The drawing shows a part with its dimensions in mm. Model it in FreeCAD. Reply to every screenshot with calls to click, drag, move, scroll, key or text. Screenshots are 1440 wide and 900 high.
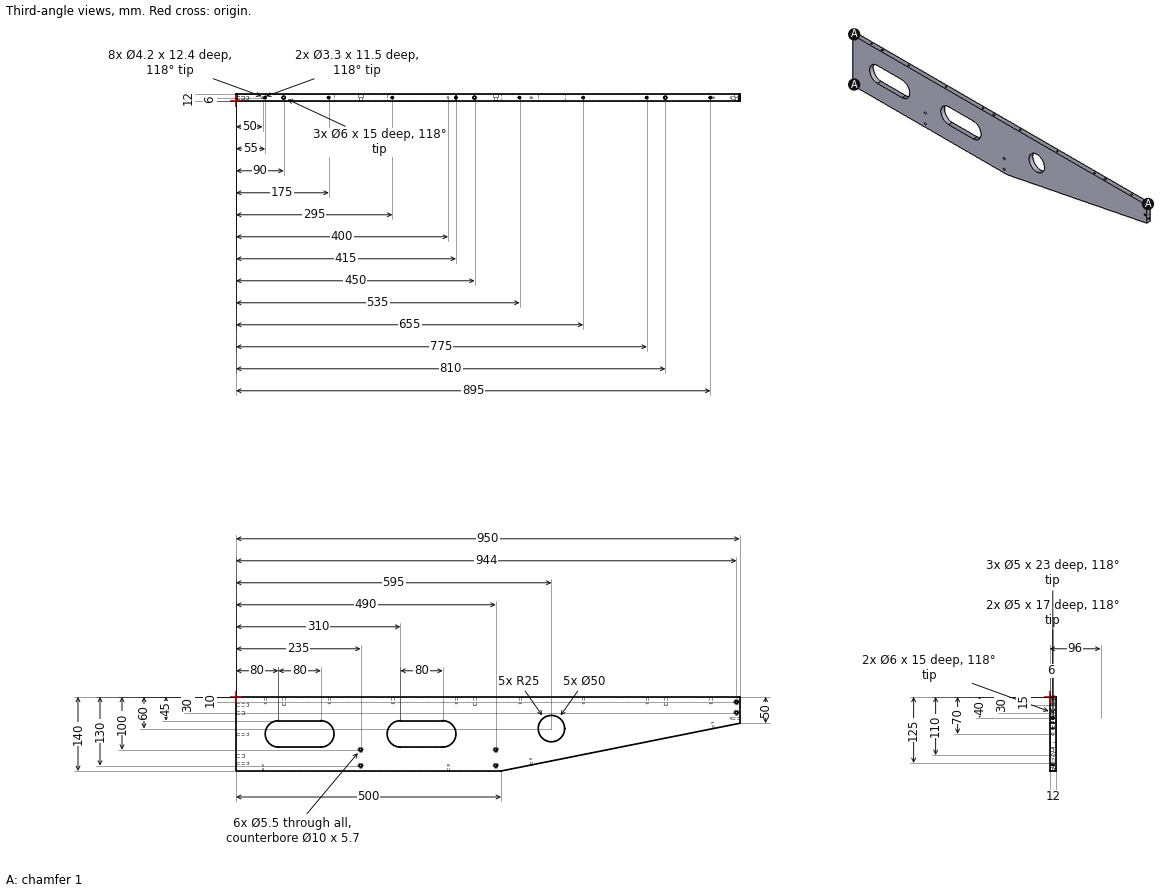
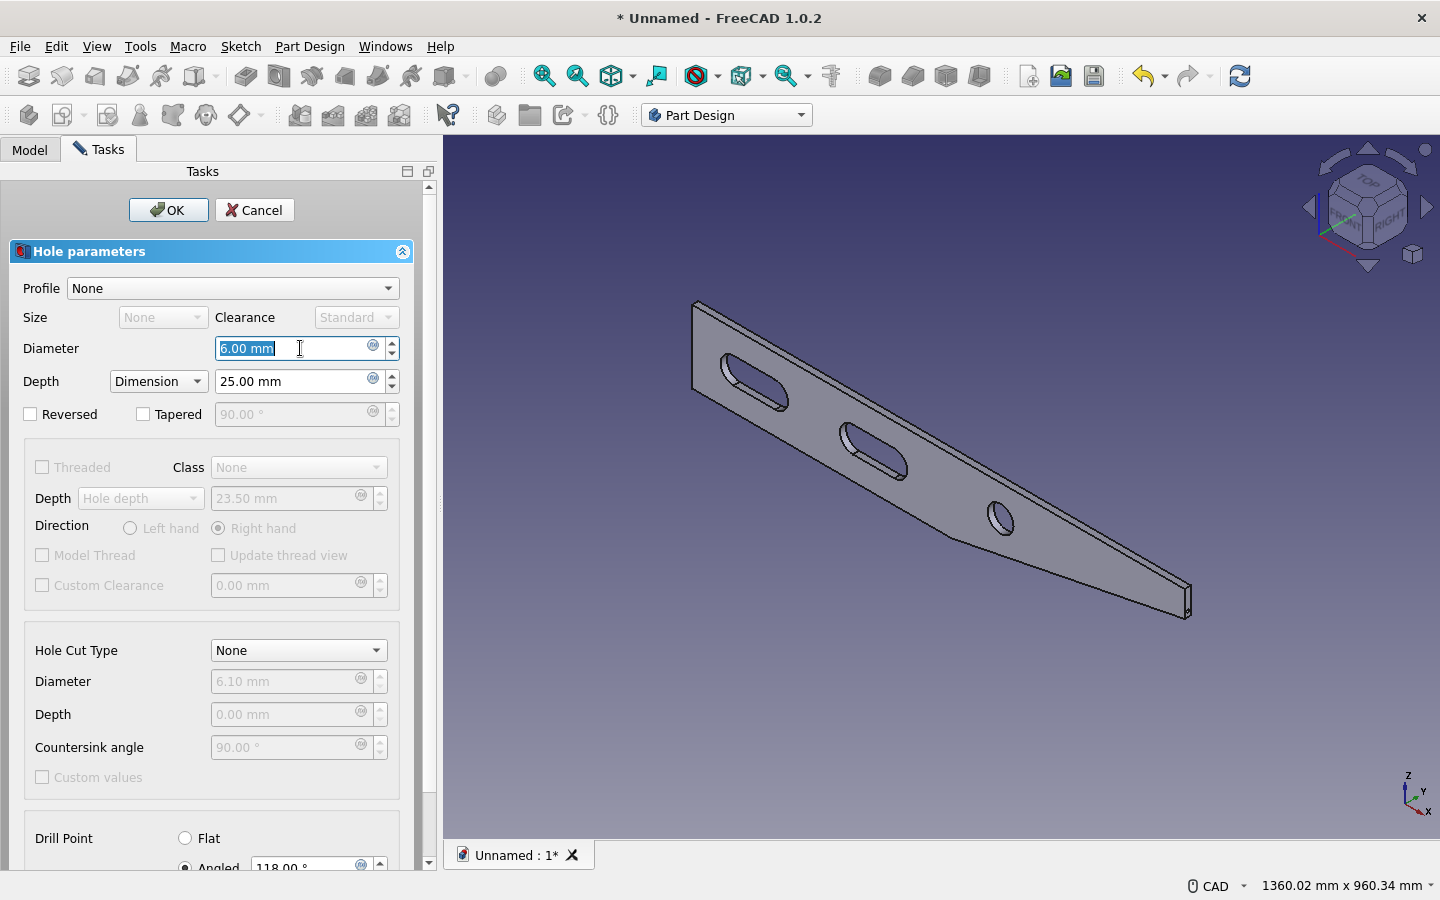
text(5)
key(Tab)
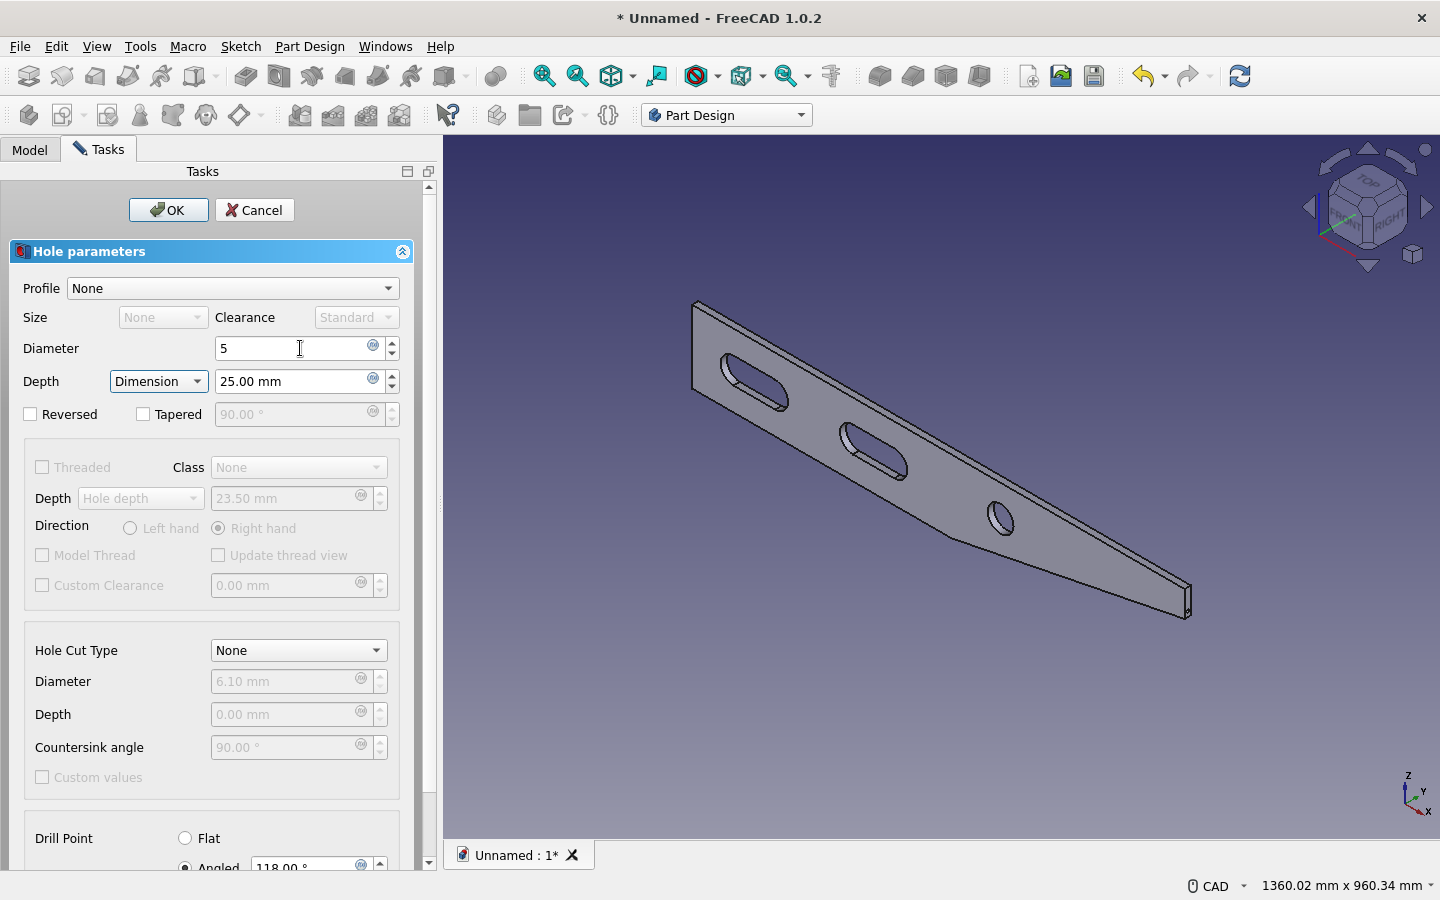
triple_click(300, 382)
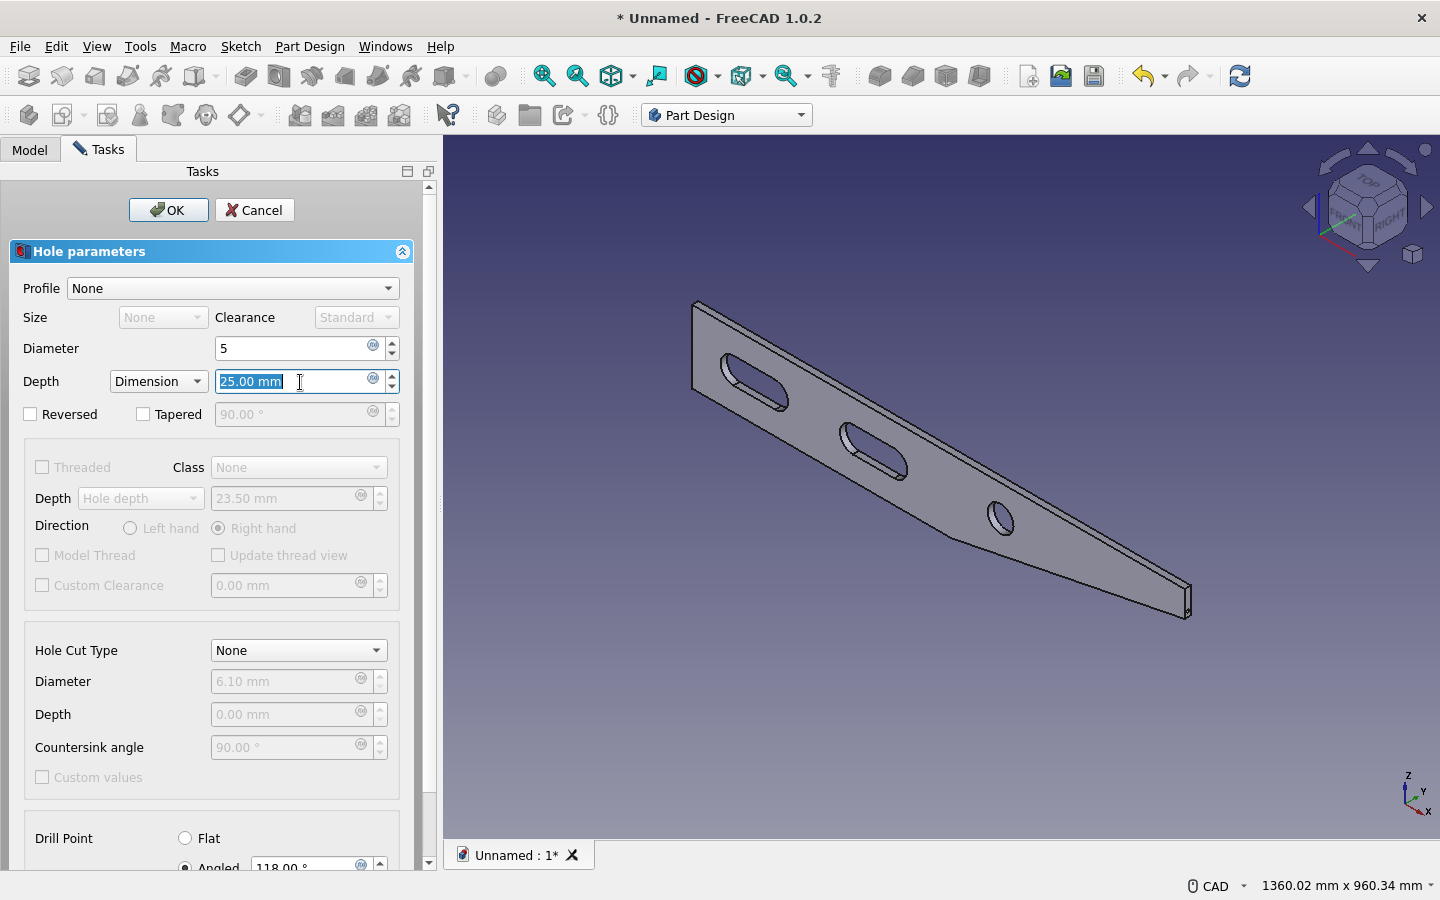
text(23)
key(Tab)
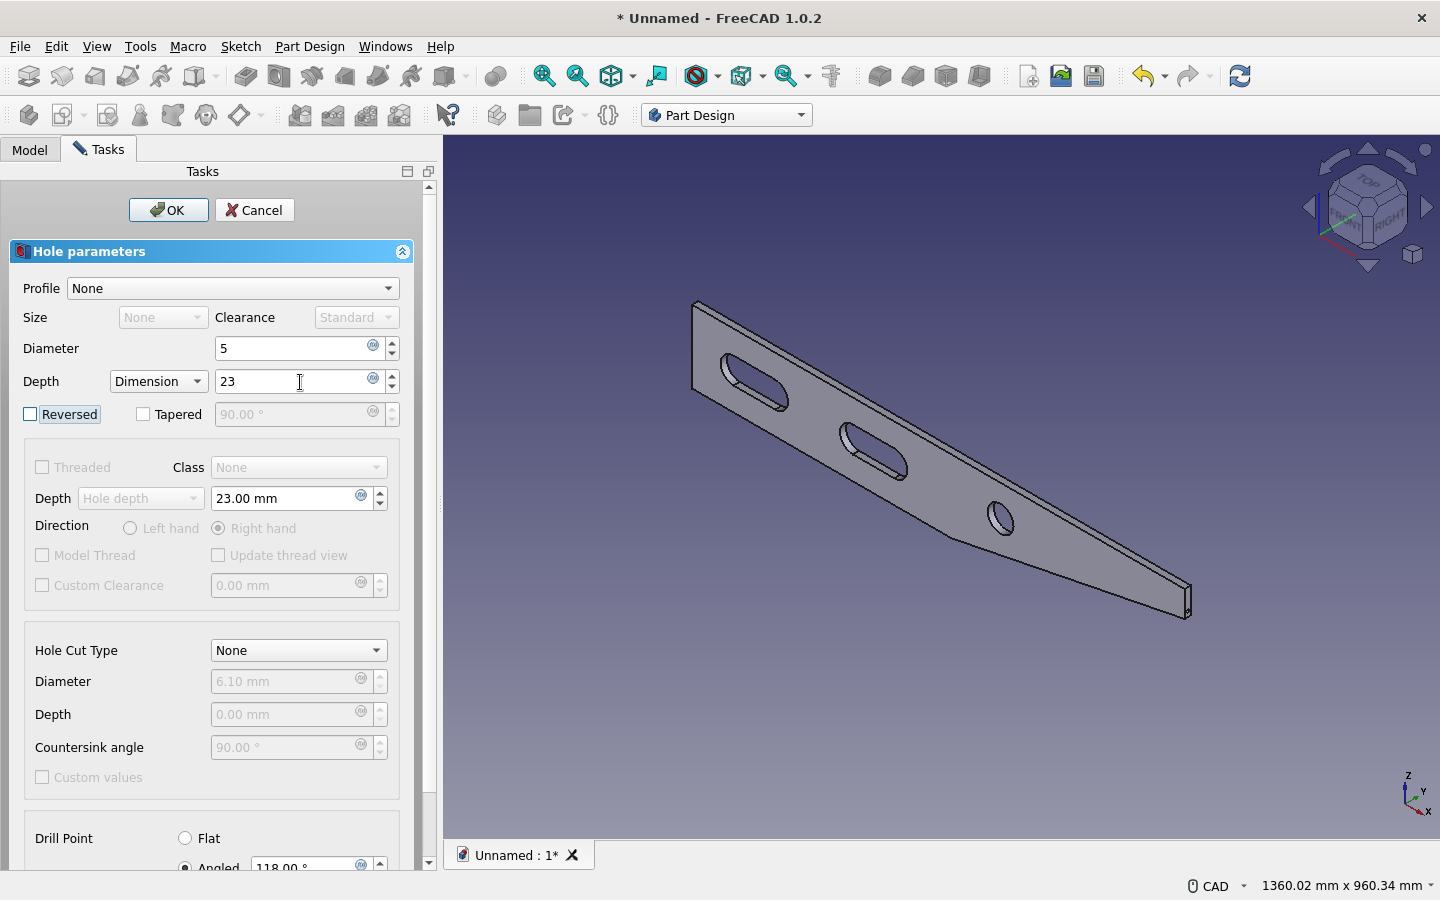
click(31, 414)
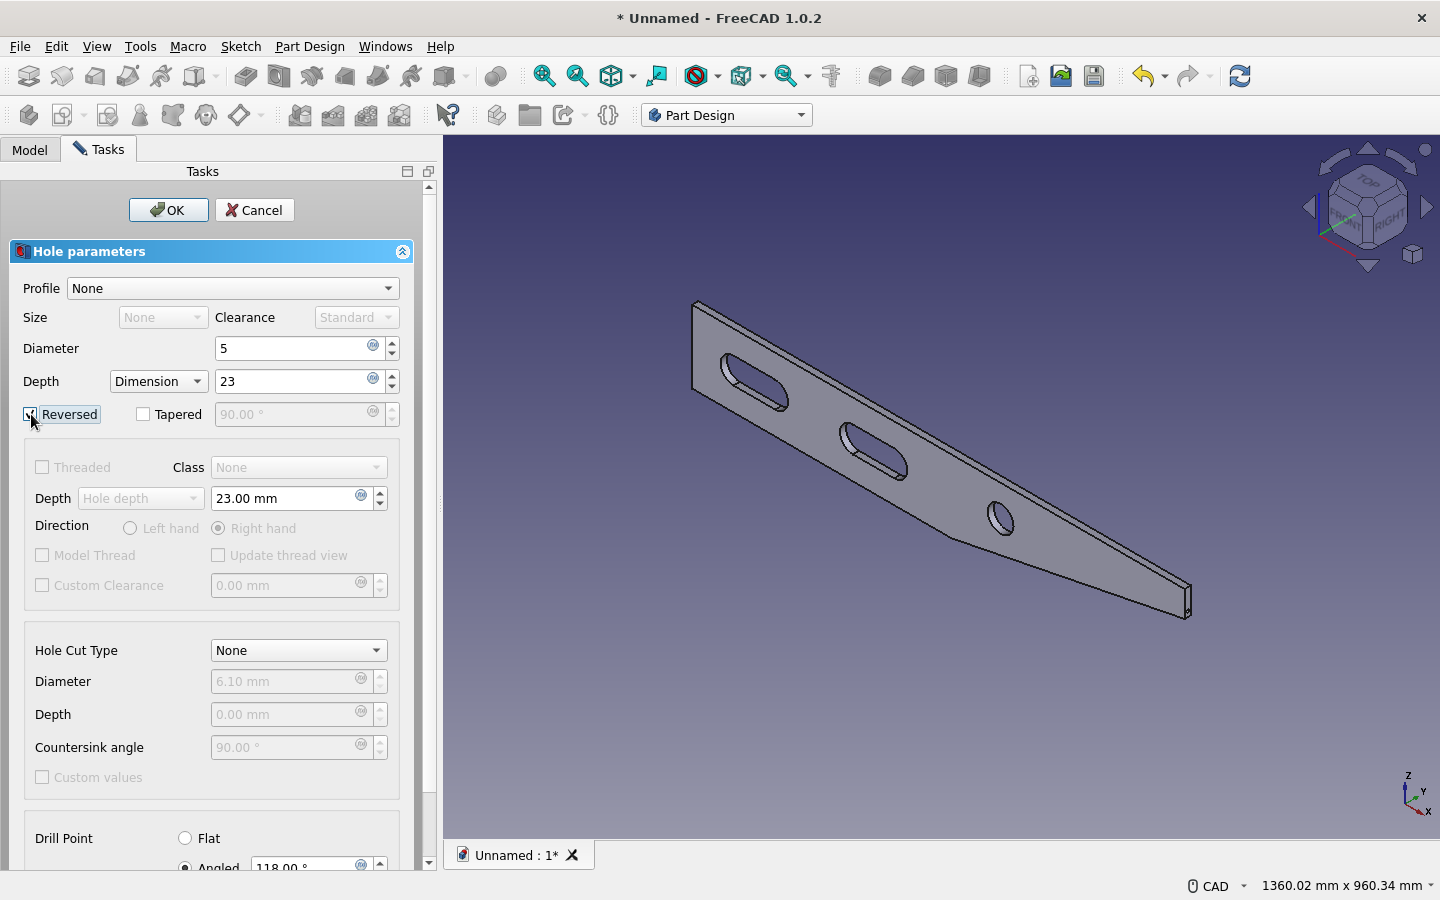
click(169, 210)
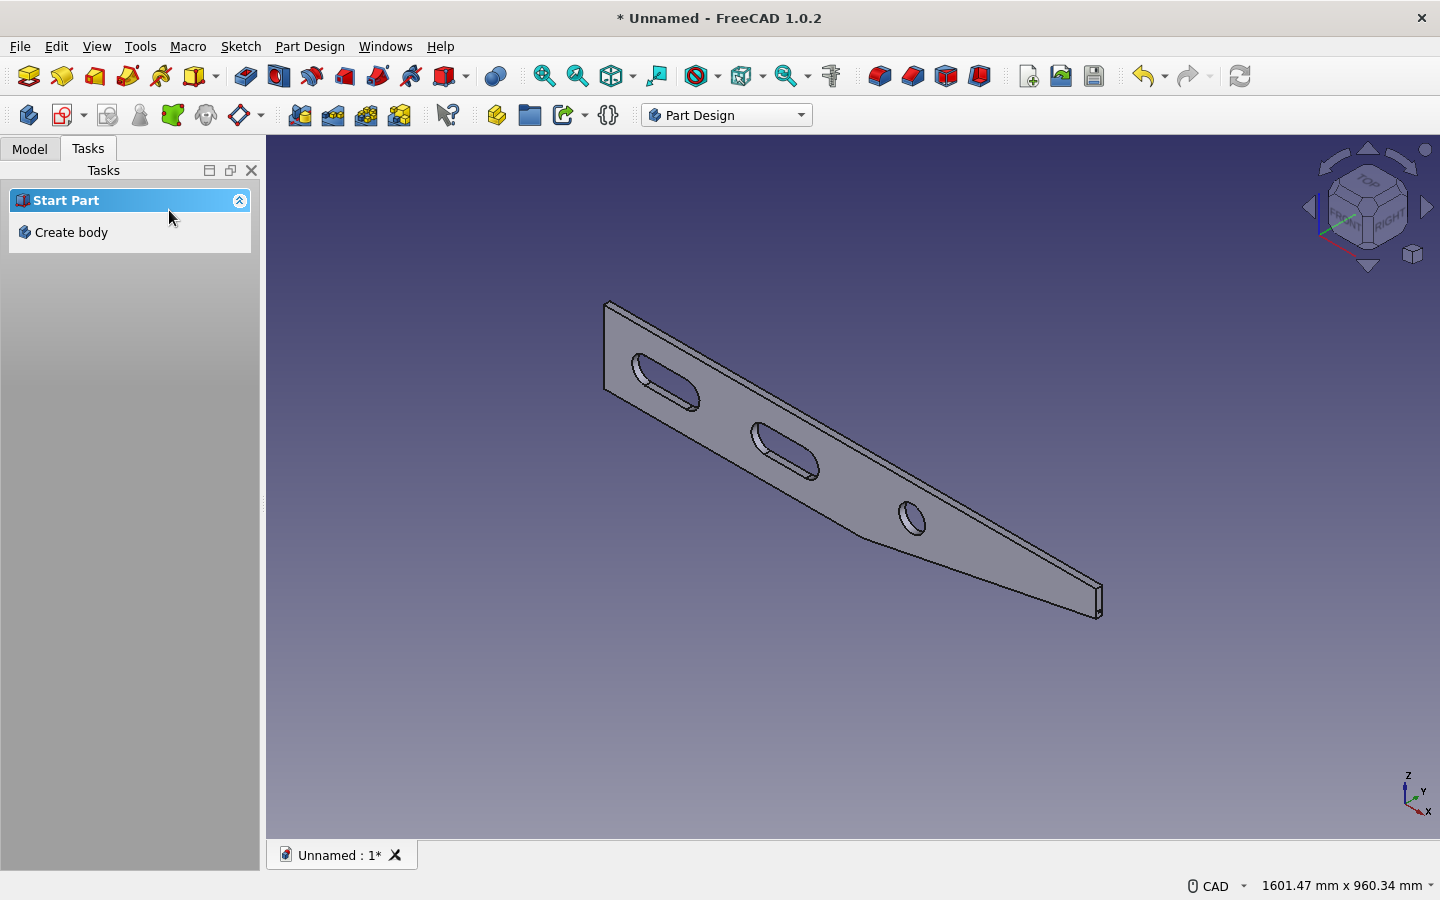
key(6)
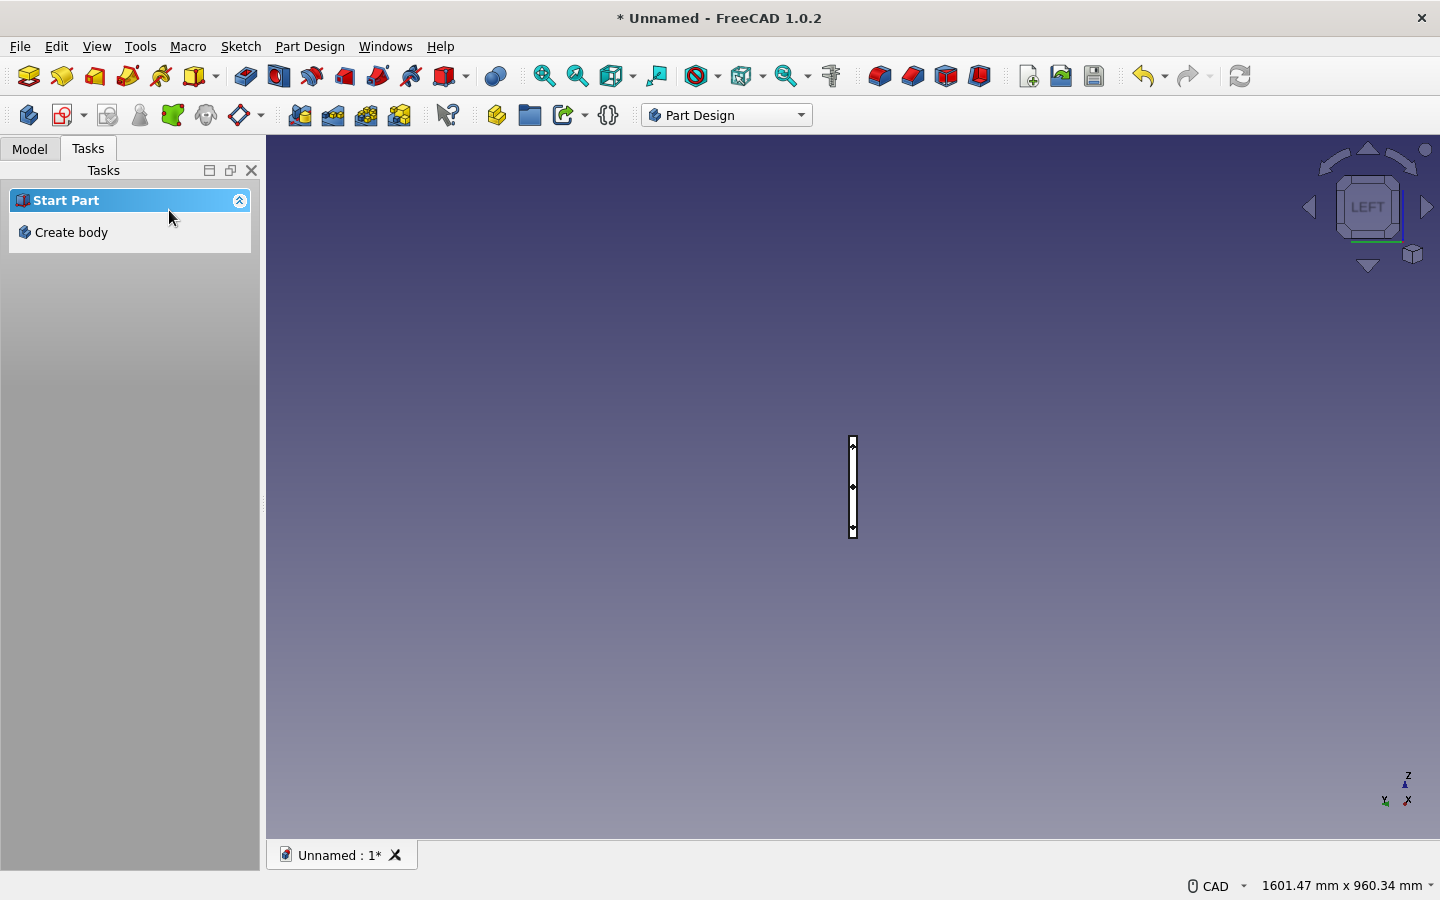
click(545, 76)